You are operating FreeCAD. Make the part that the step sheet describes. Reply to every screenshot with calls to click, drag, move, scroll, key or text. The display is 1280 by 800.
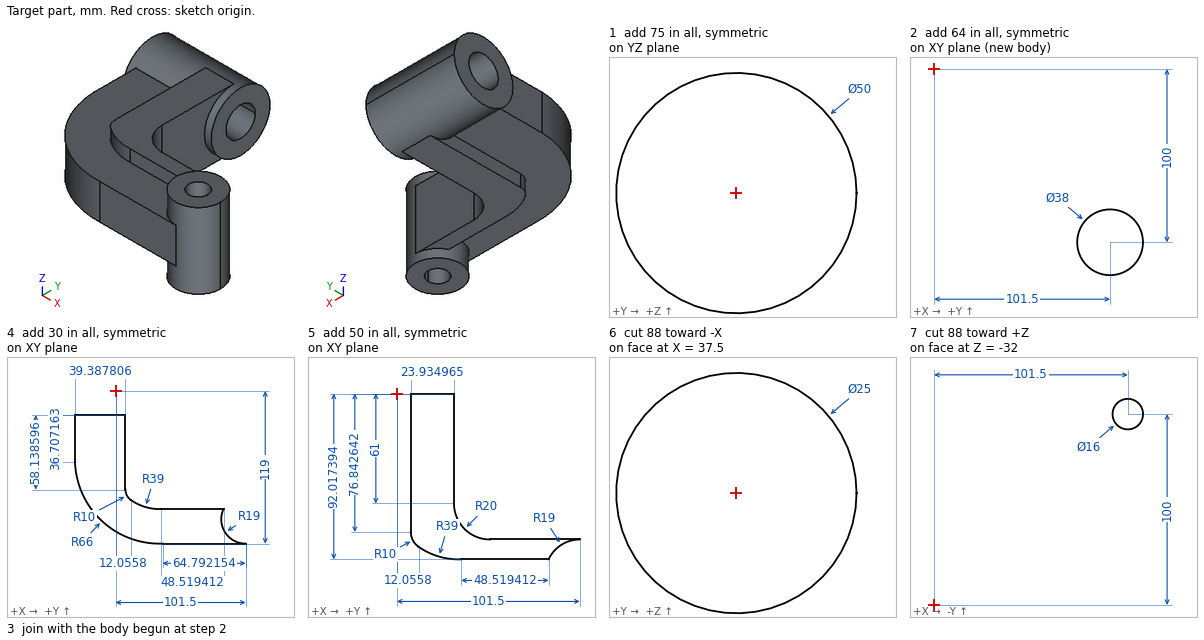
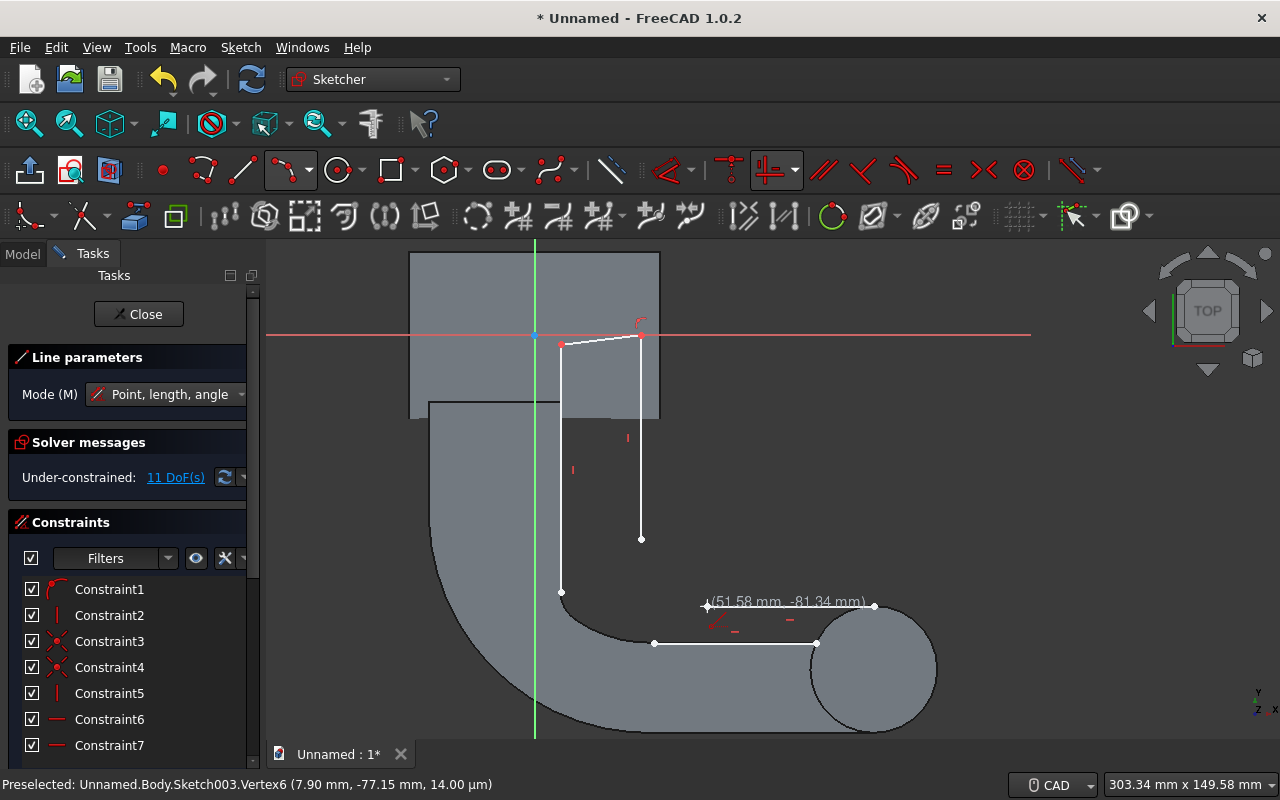
click(284, 170)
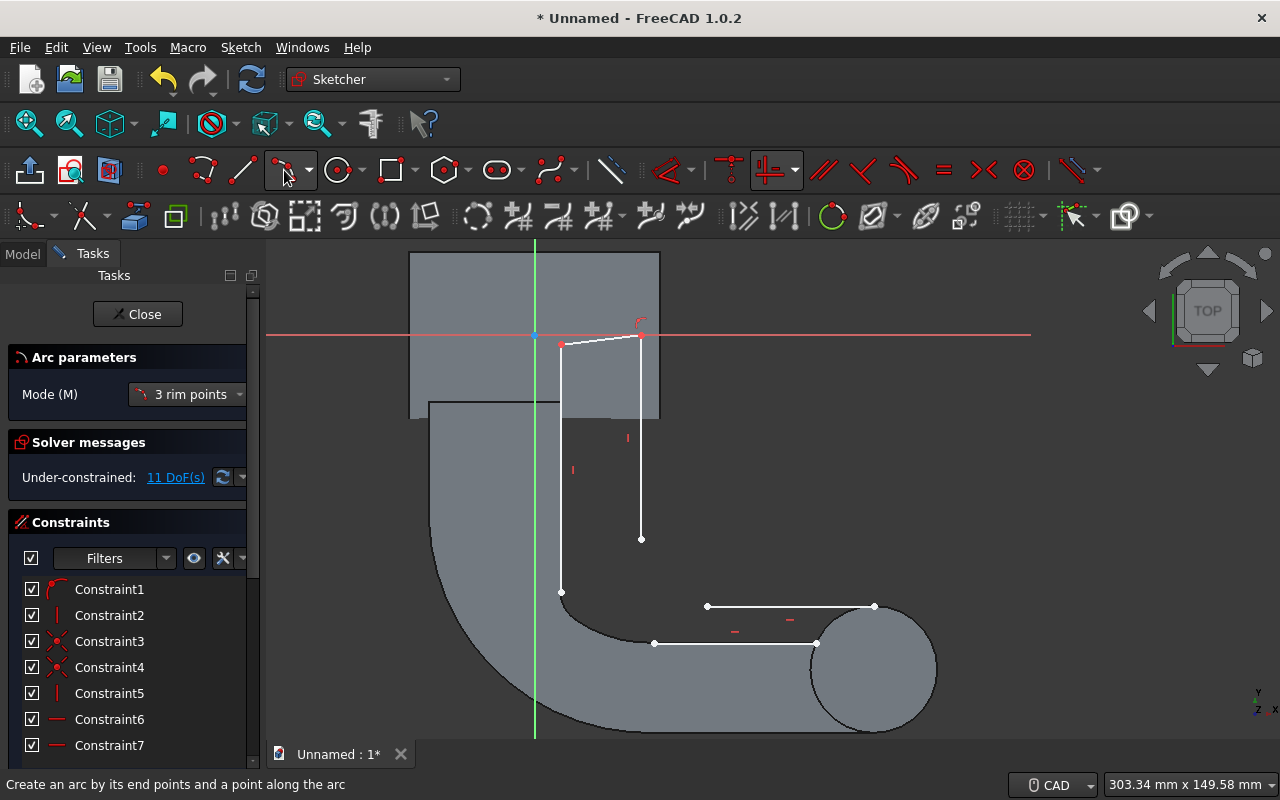
click(561, 593)
click(575, 619)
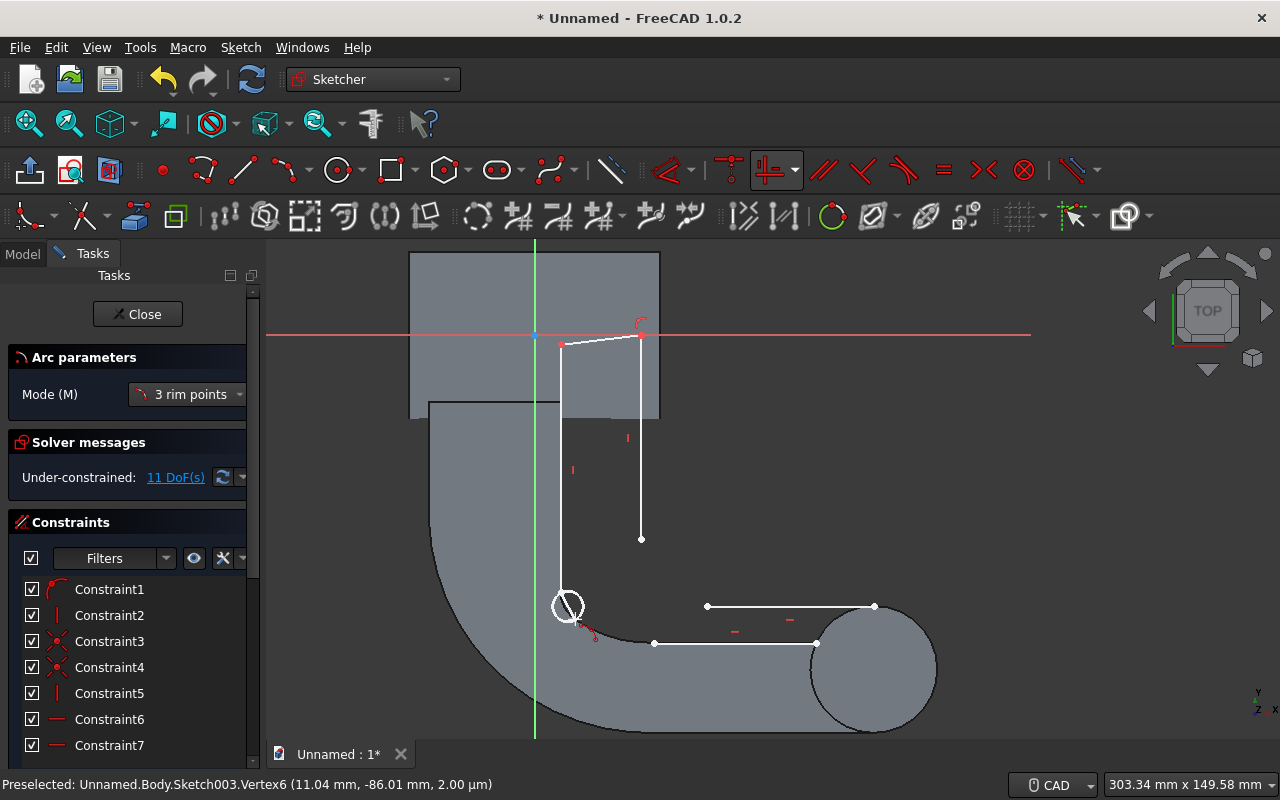
scroll(564, 607, up, 8)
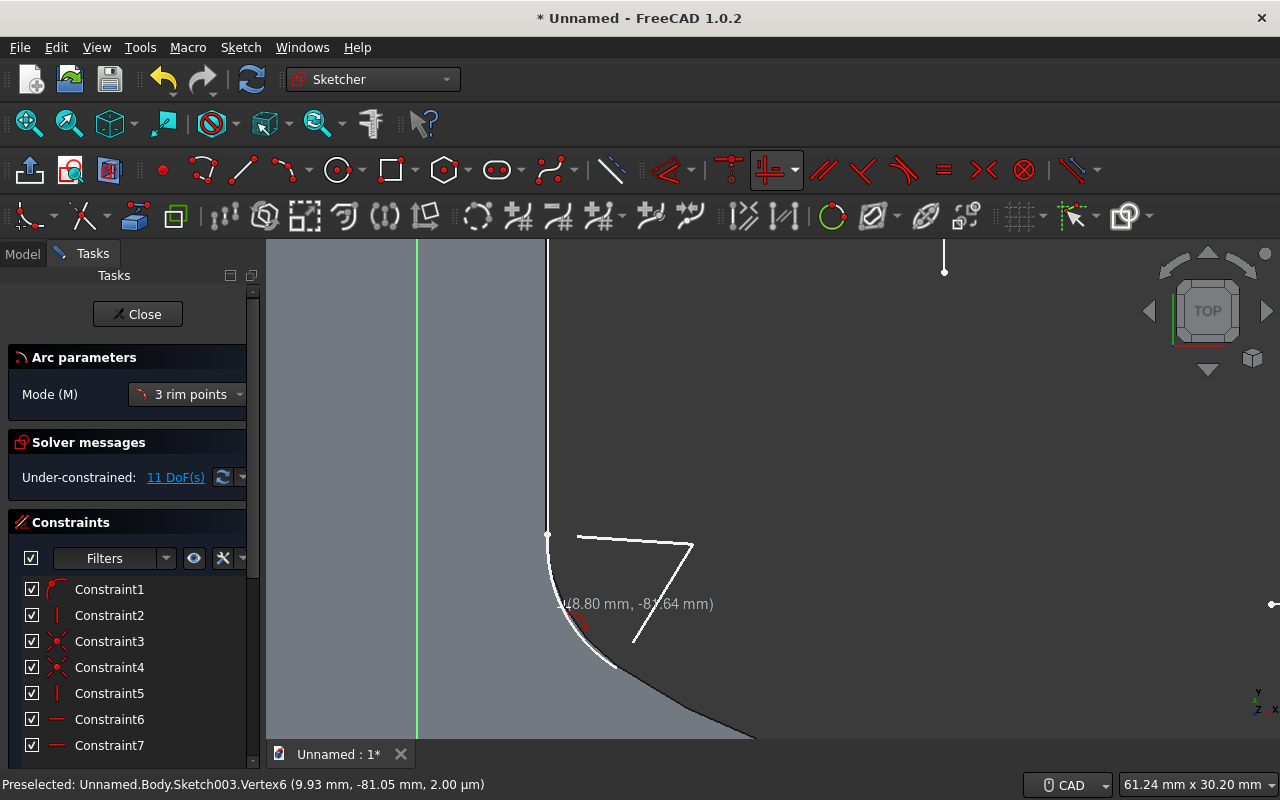
click(565, 606)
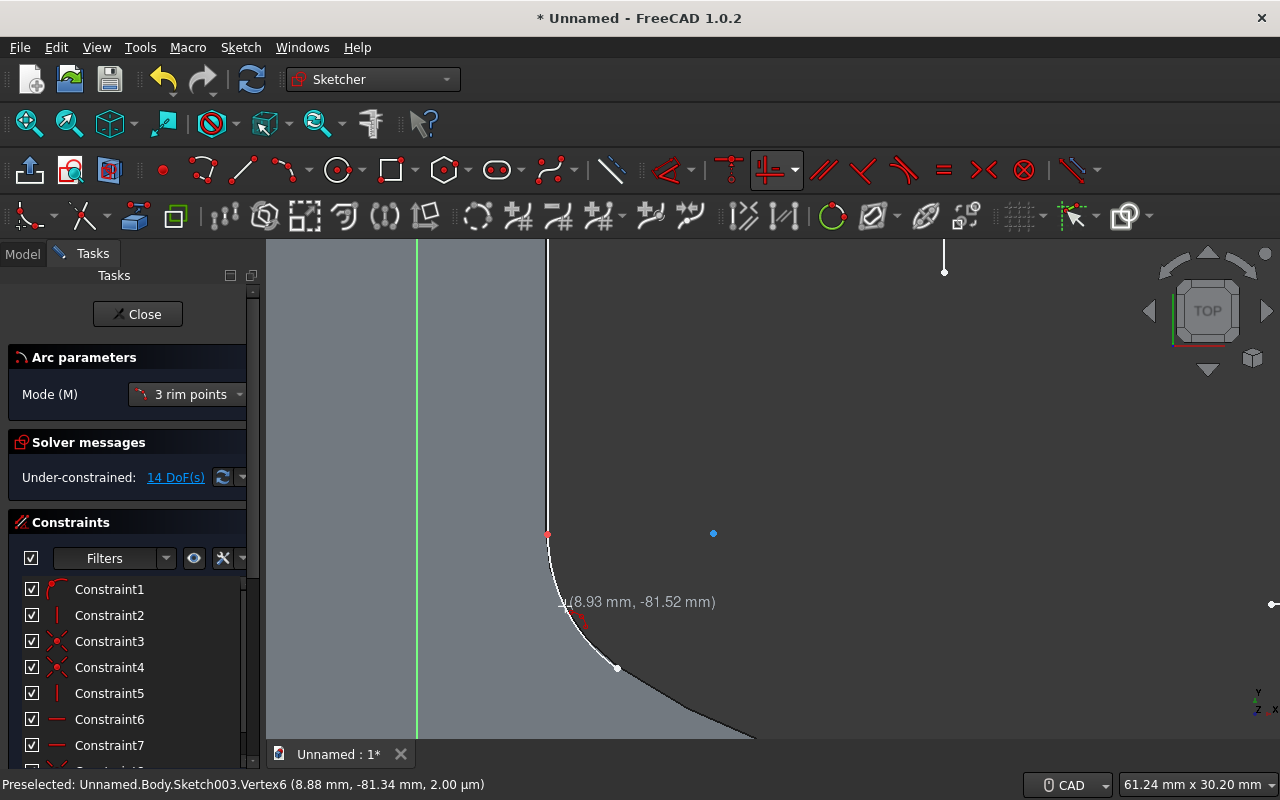
scroll(565, 608, down, 8)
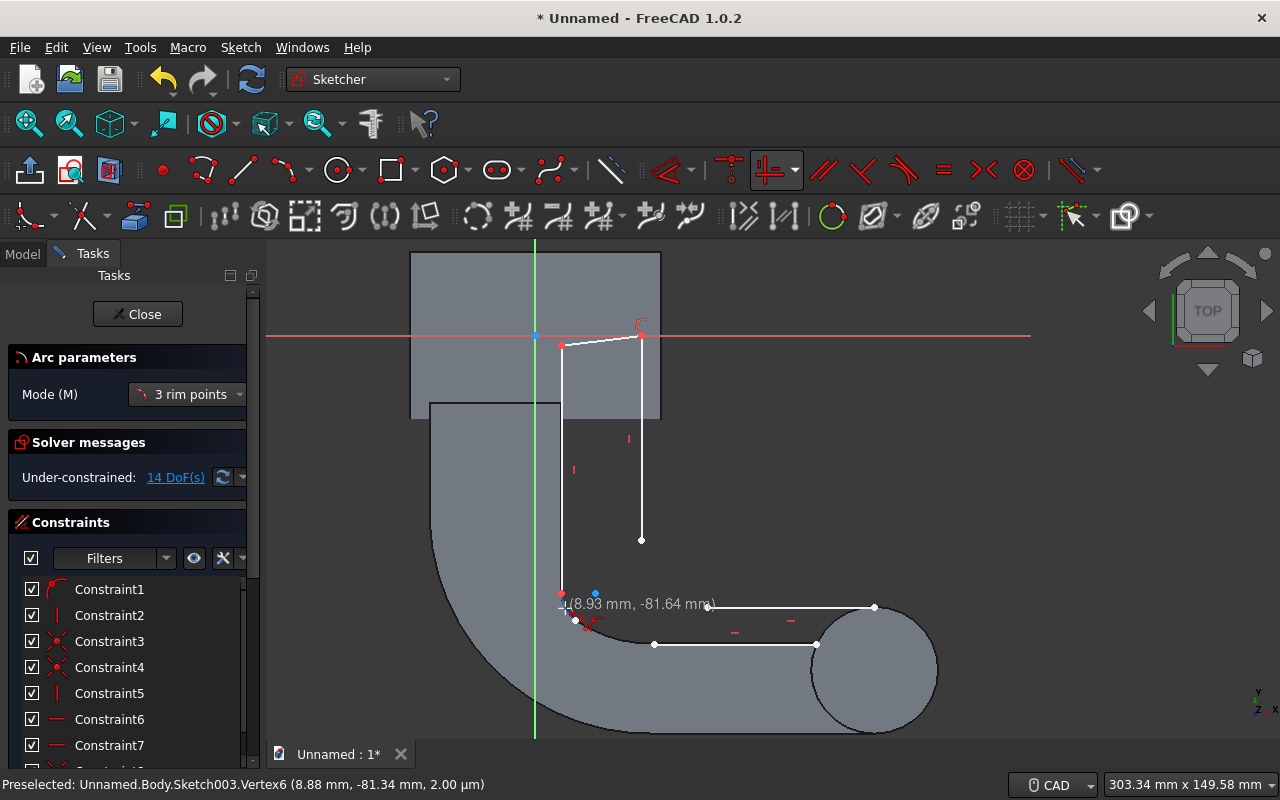
click(576, 621)
click(655, 645)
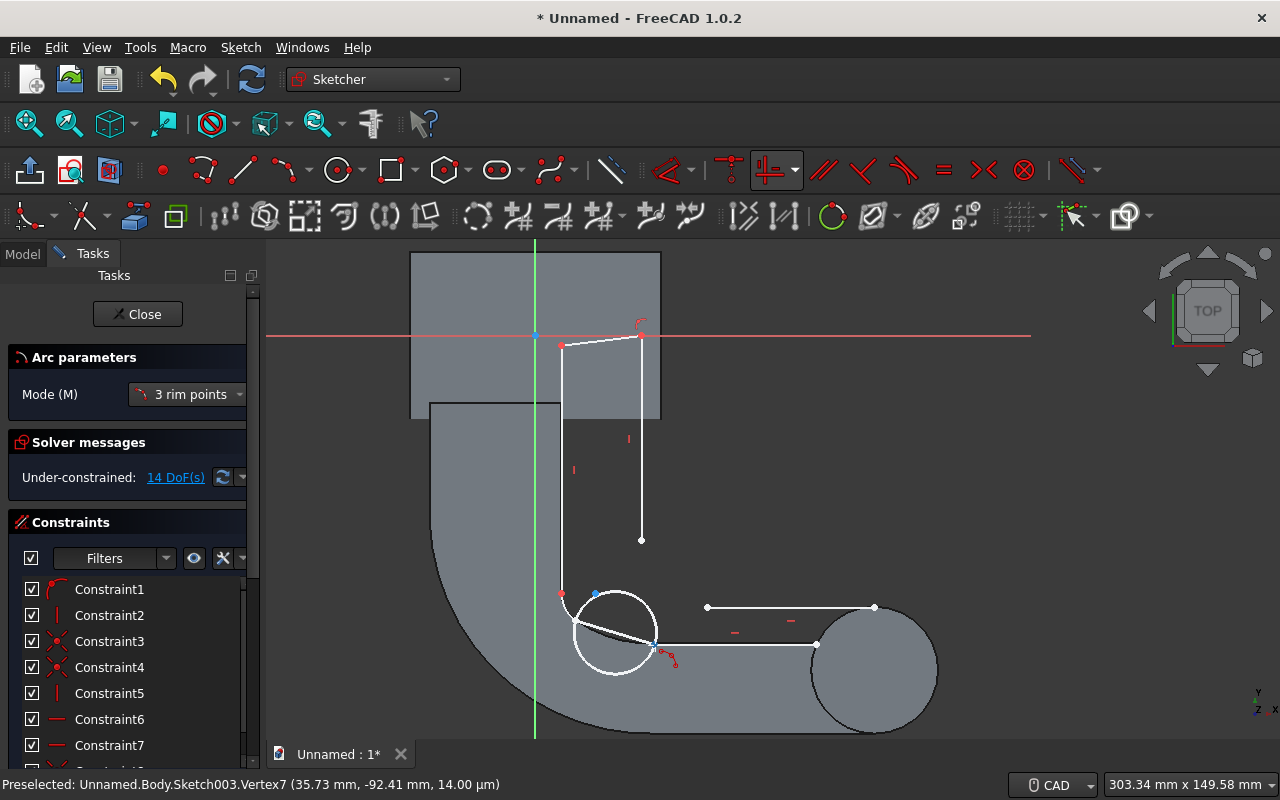
scroll(613, 638, up, 5)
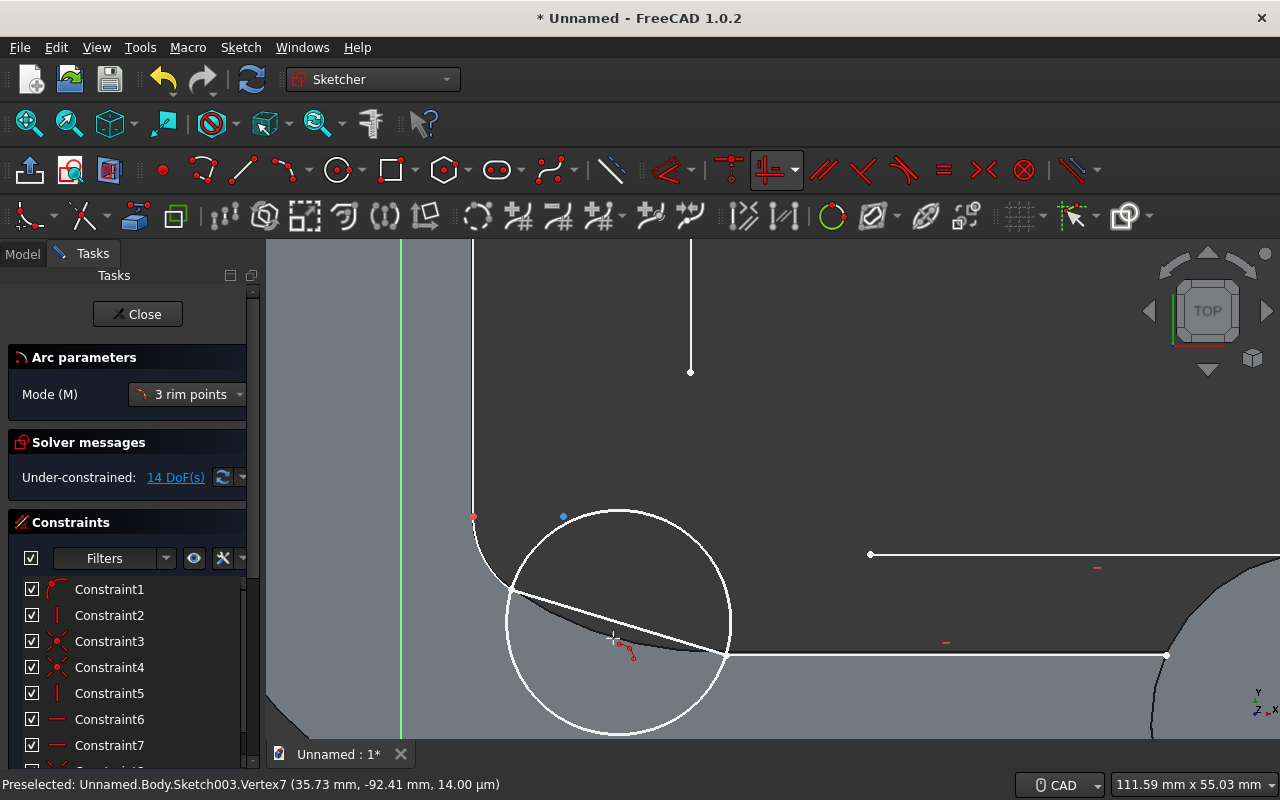
click(613, 637)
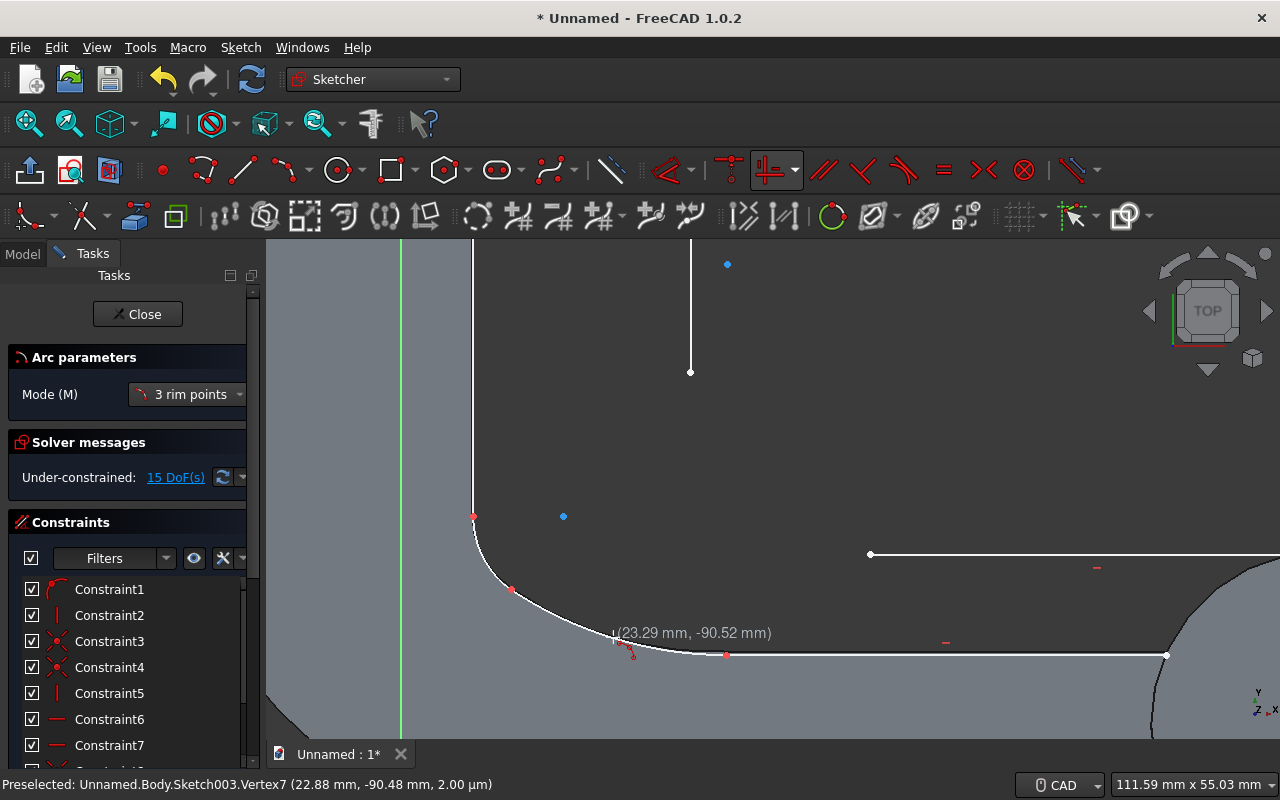
scroll(613, 638, down, 5)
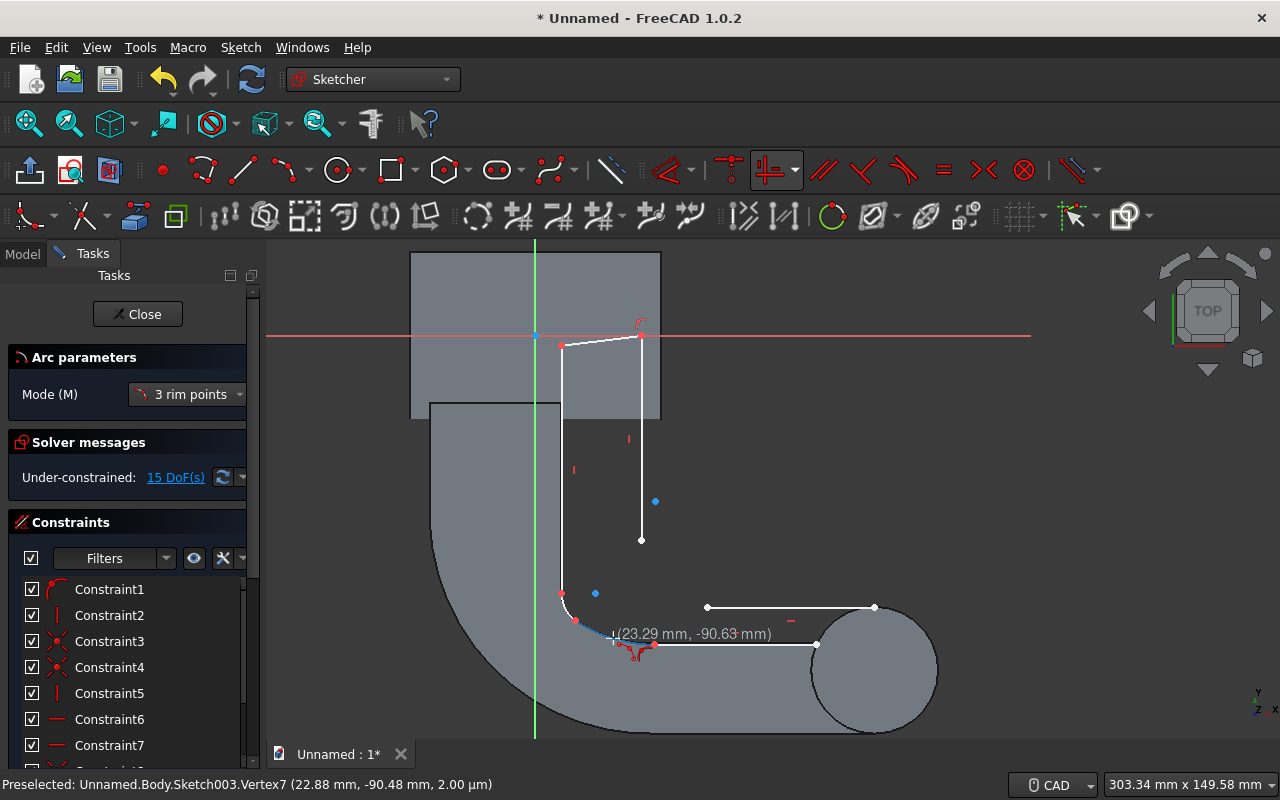
click(817, 645)
click(875, 608)